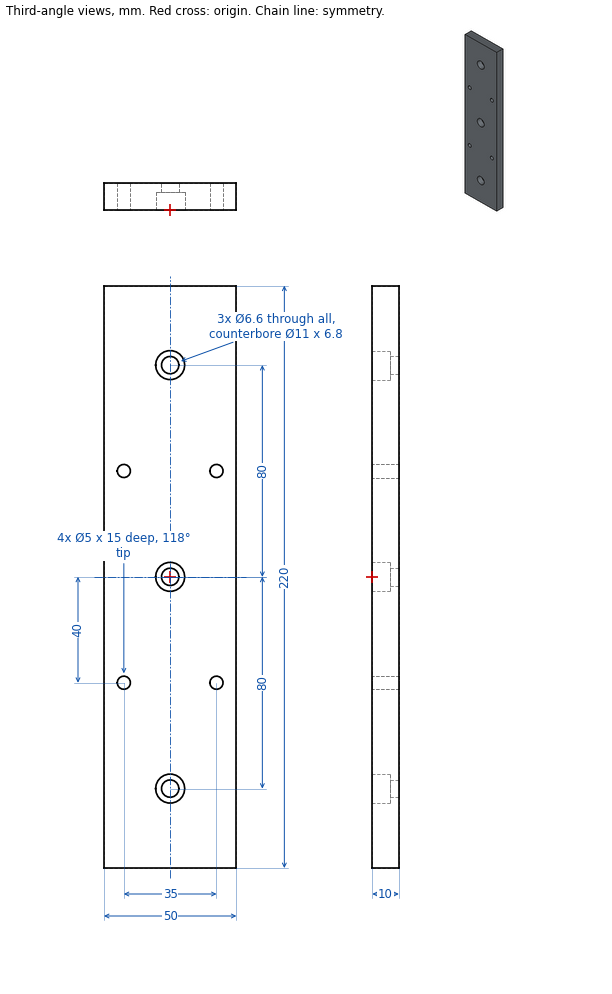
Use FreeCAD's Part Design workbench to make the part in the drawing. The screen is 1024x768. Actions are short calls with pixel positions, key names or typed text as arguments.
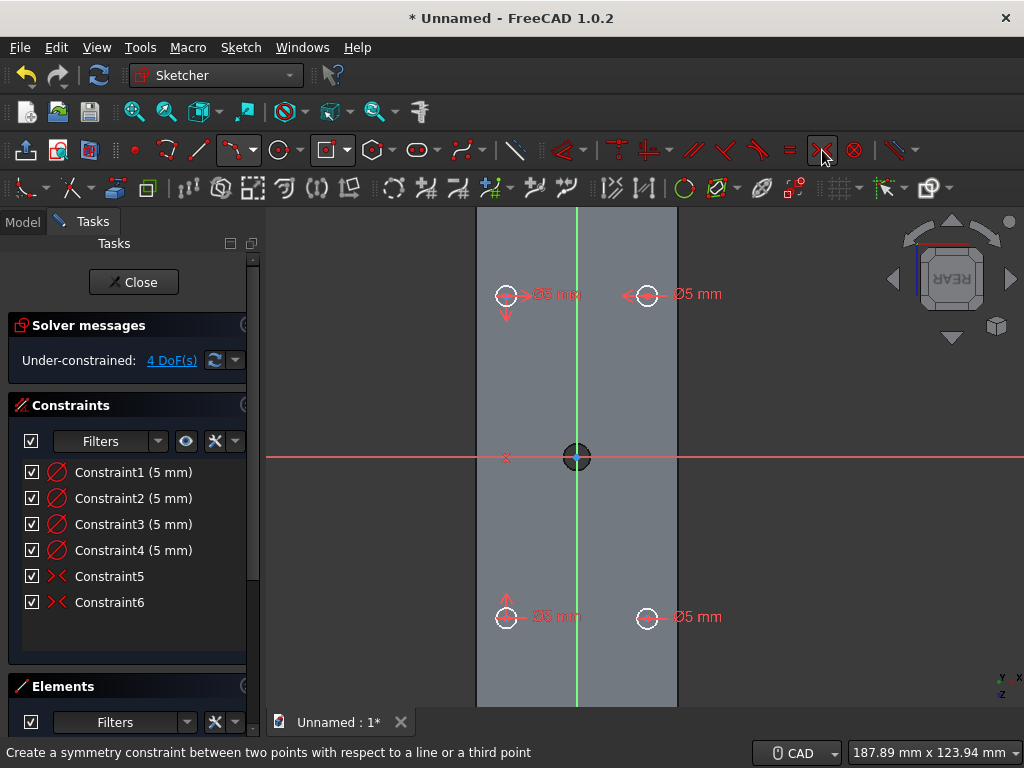
click(506, 618)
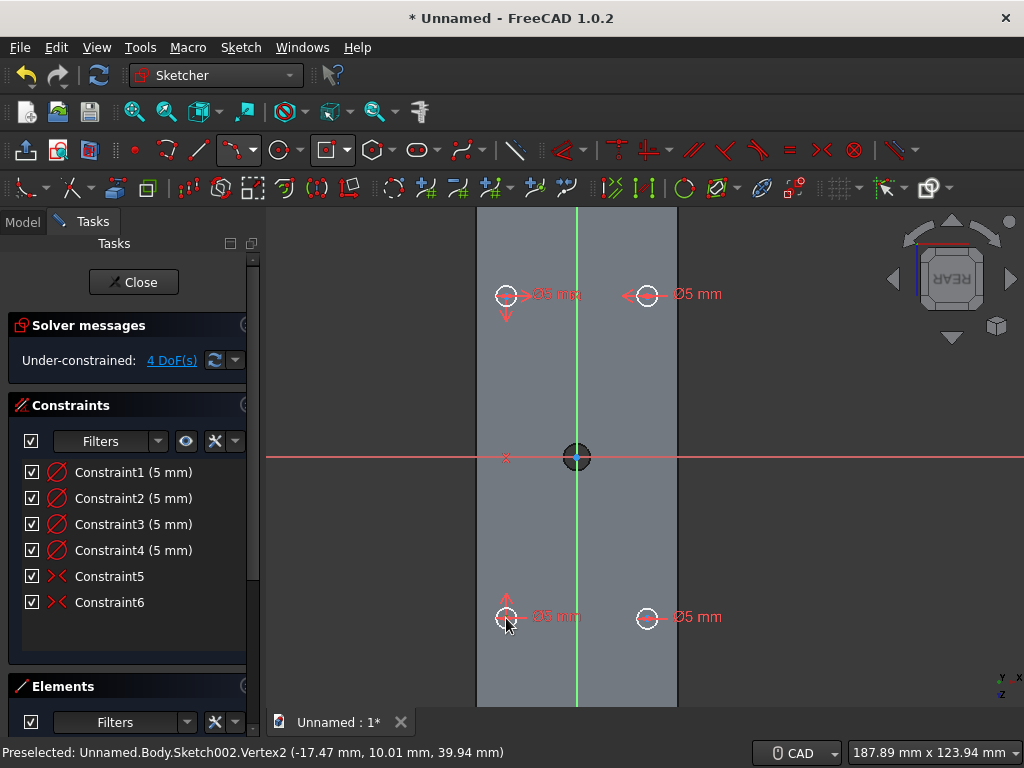
click(647, 619)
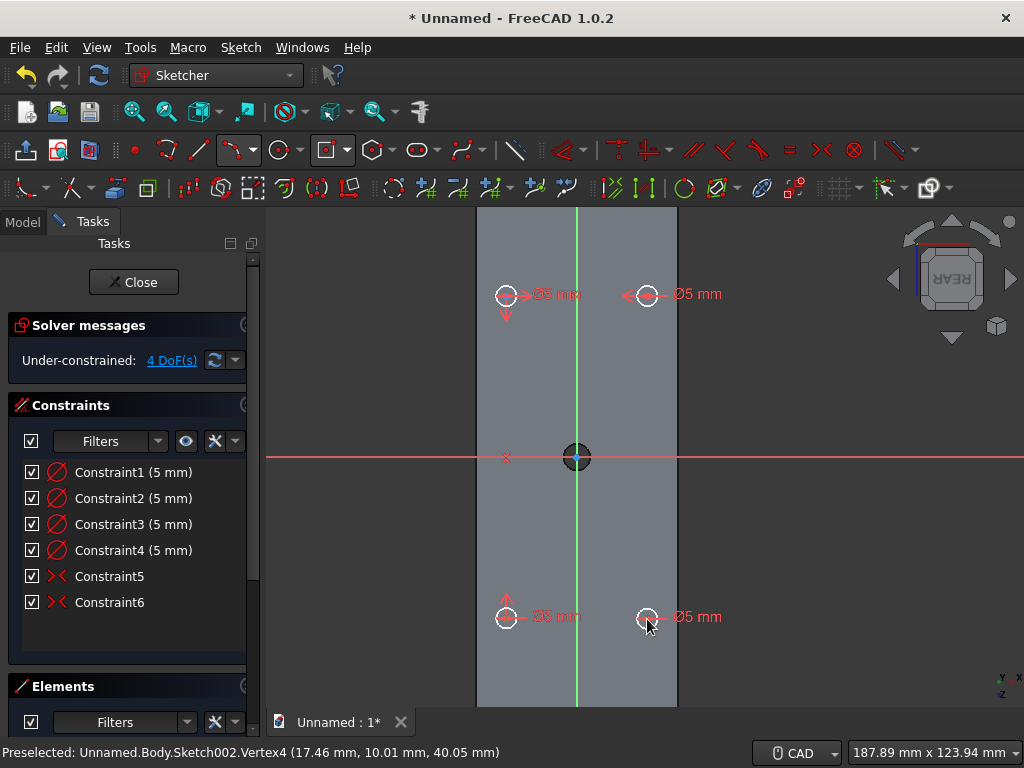
click(577, 647)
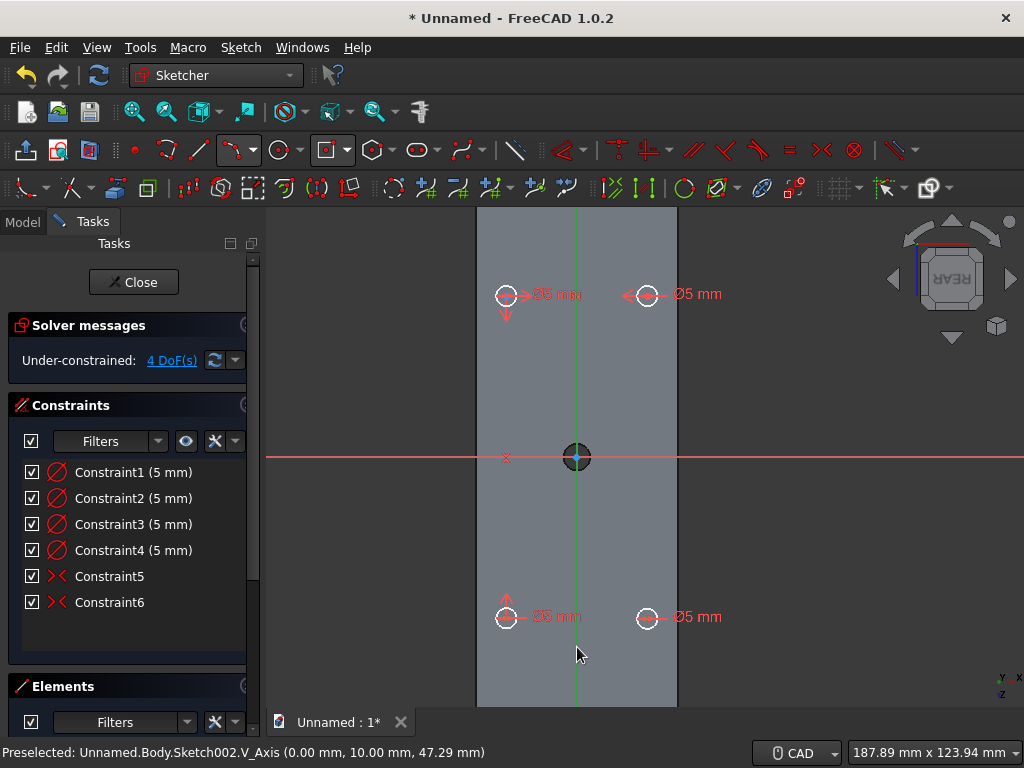
click(822, 150)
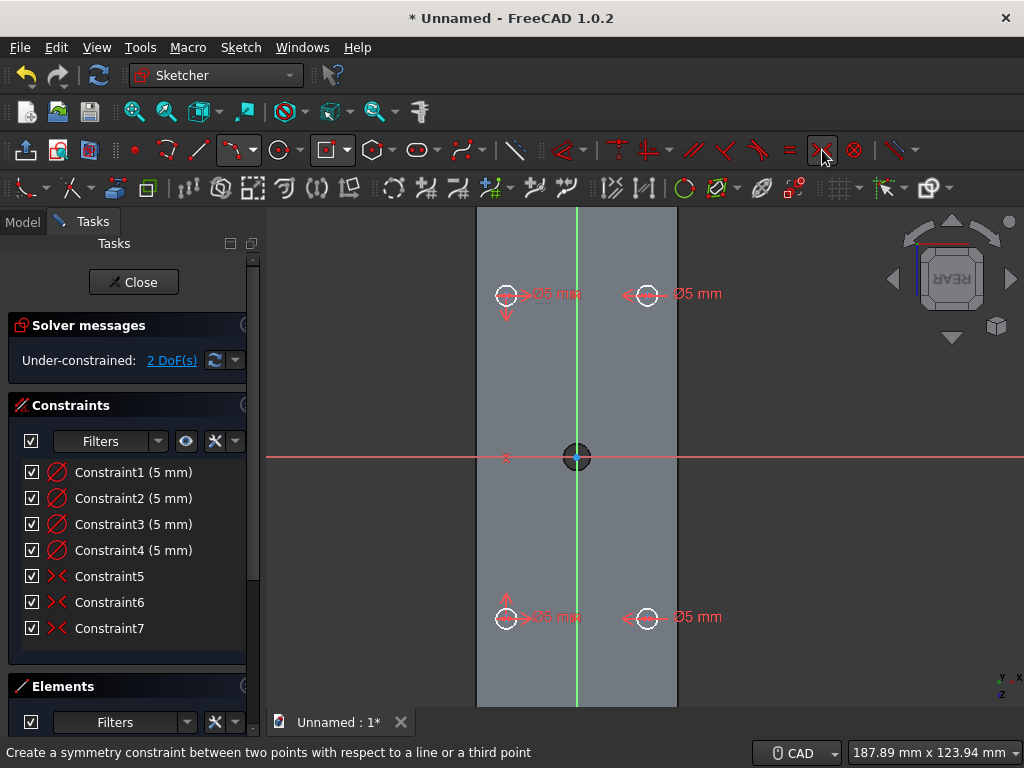
key(d)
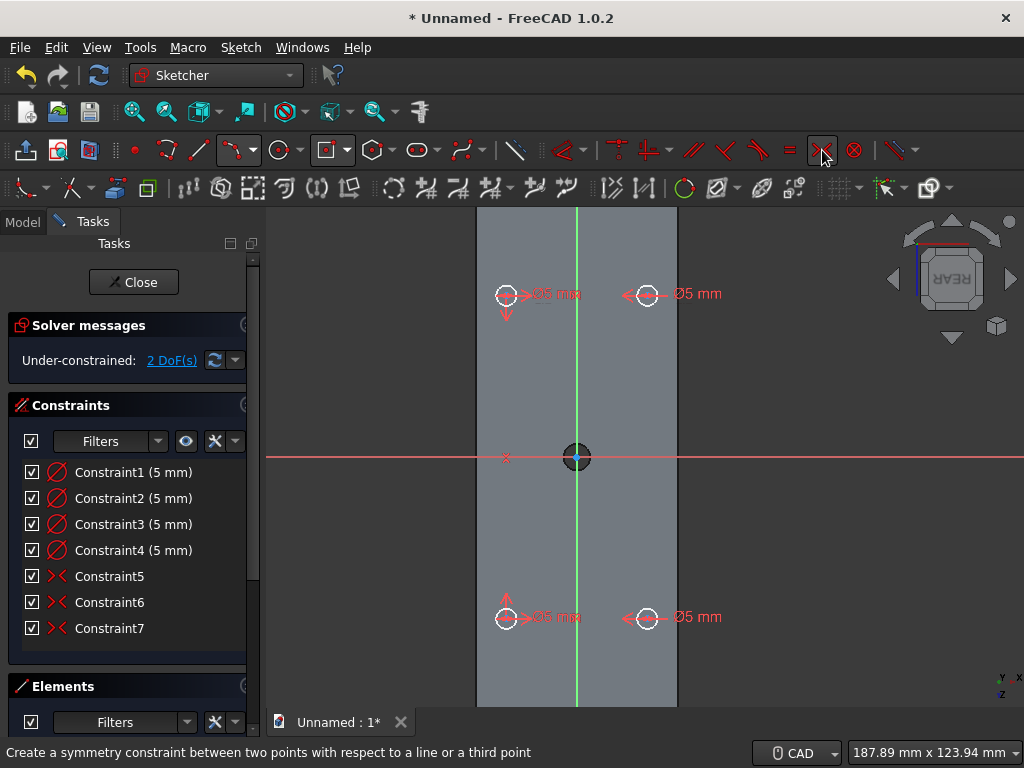
click(506, 296)
click(472, 376)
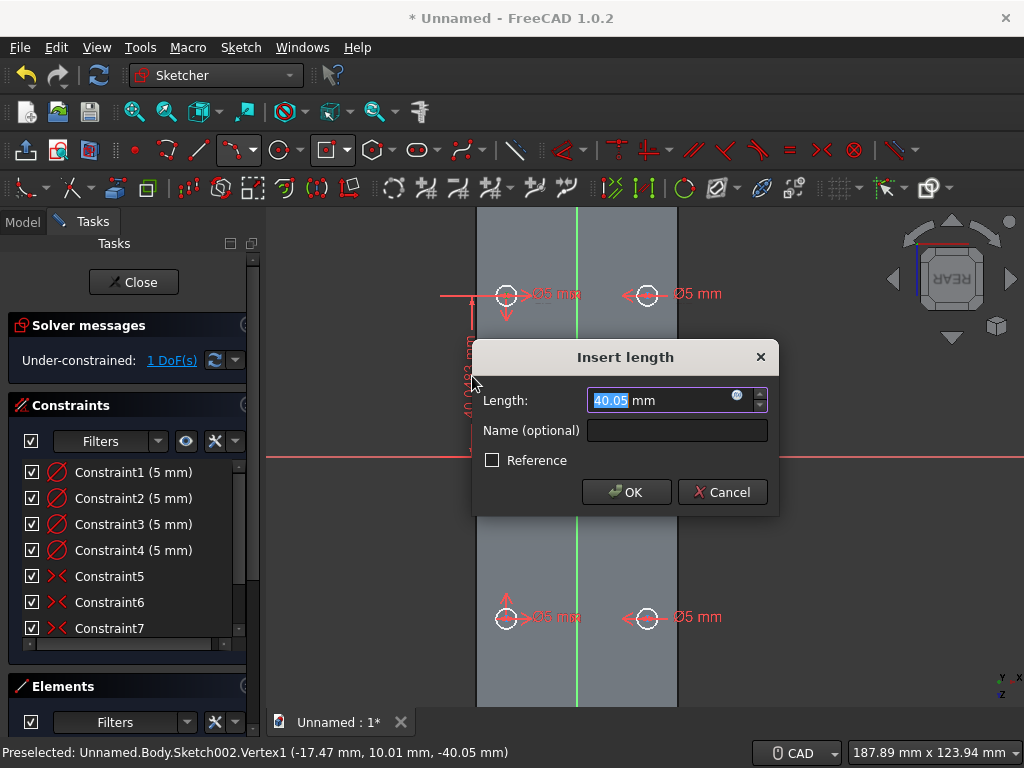
text(40)
key(Return)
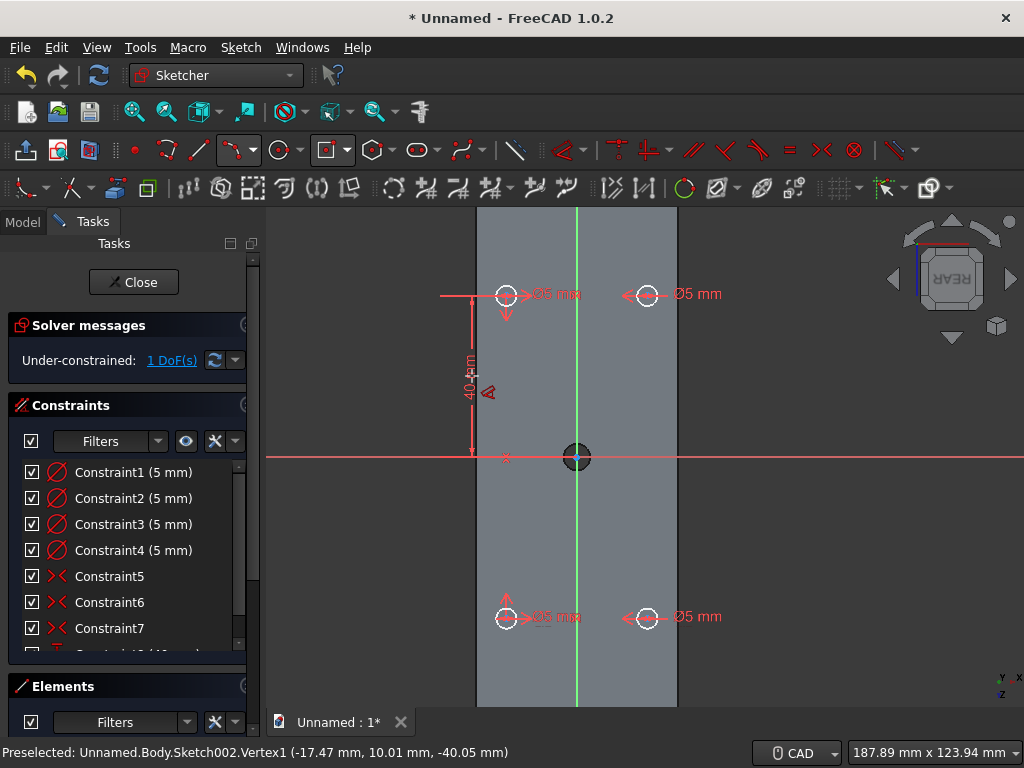
click(506, 296)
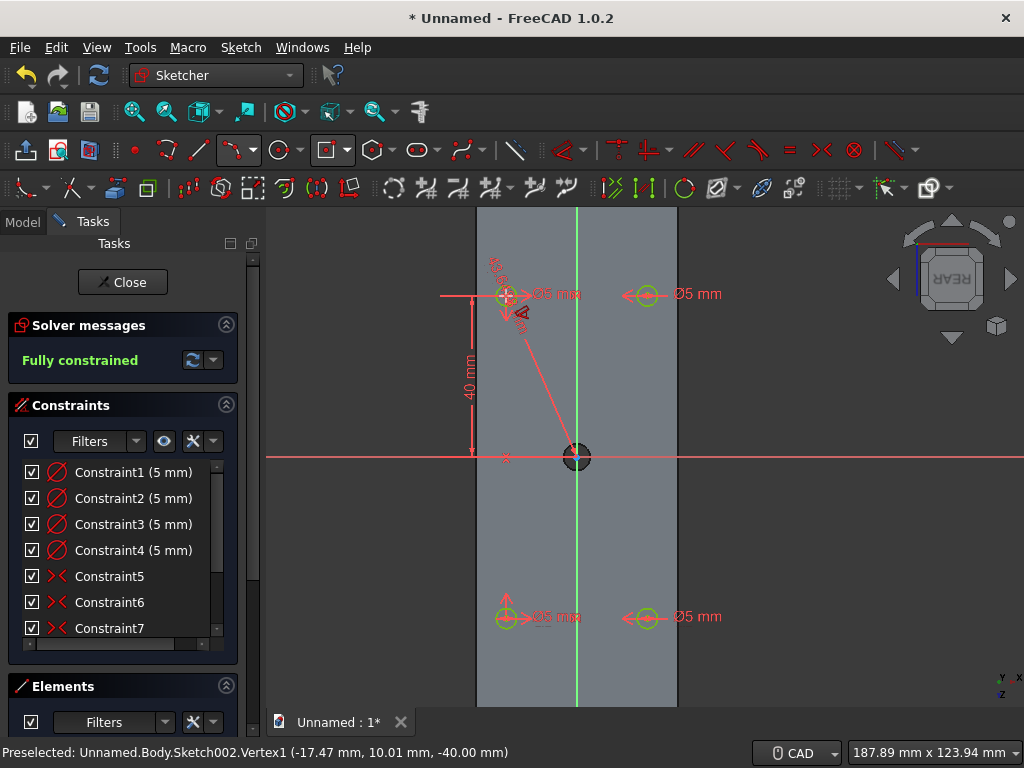
click(647, 296)
click(544, 262)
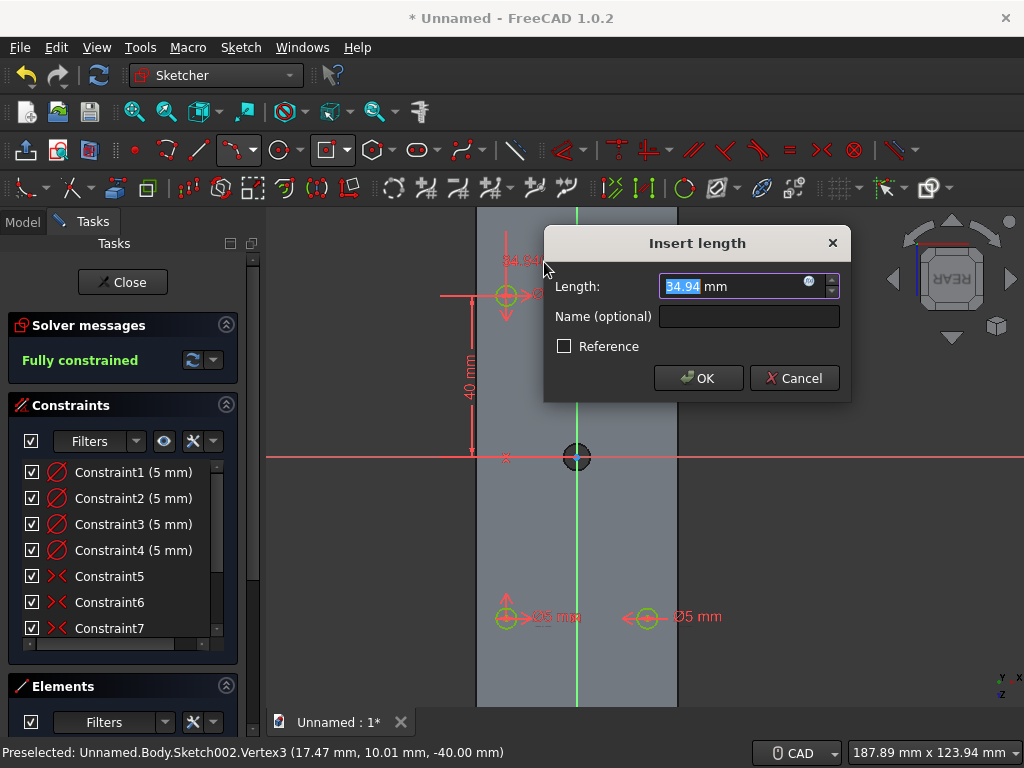
text(35)
key(Return)
key(Escape)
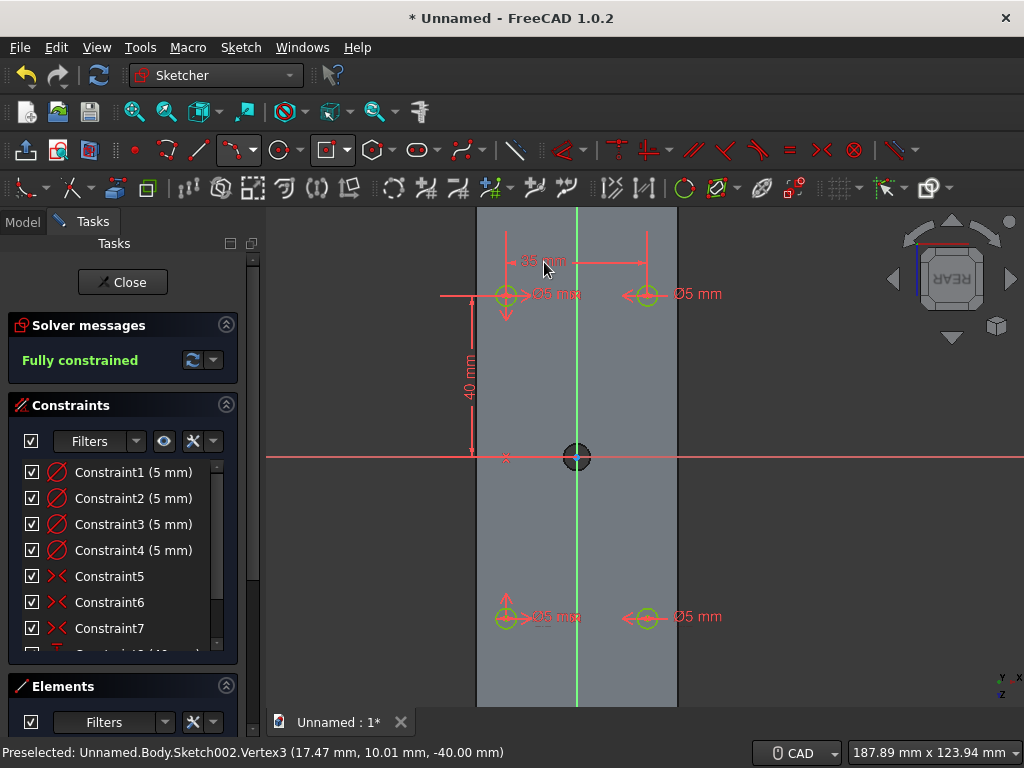
click(123, 282)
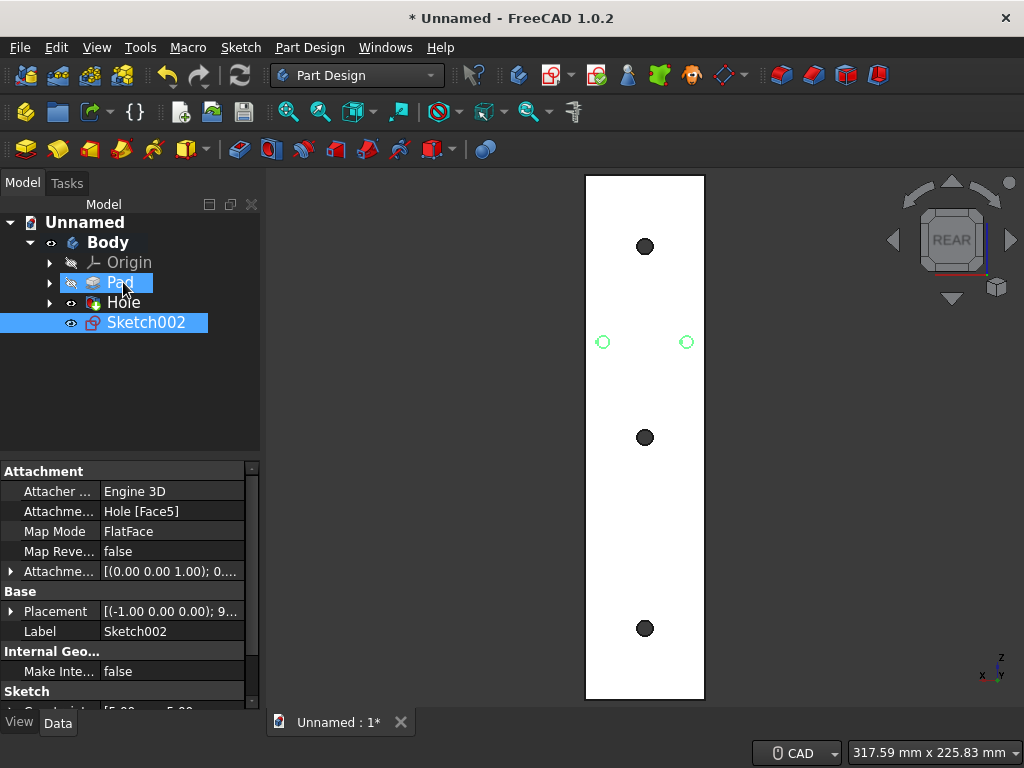
click(272, 150)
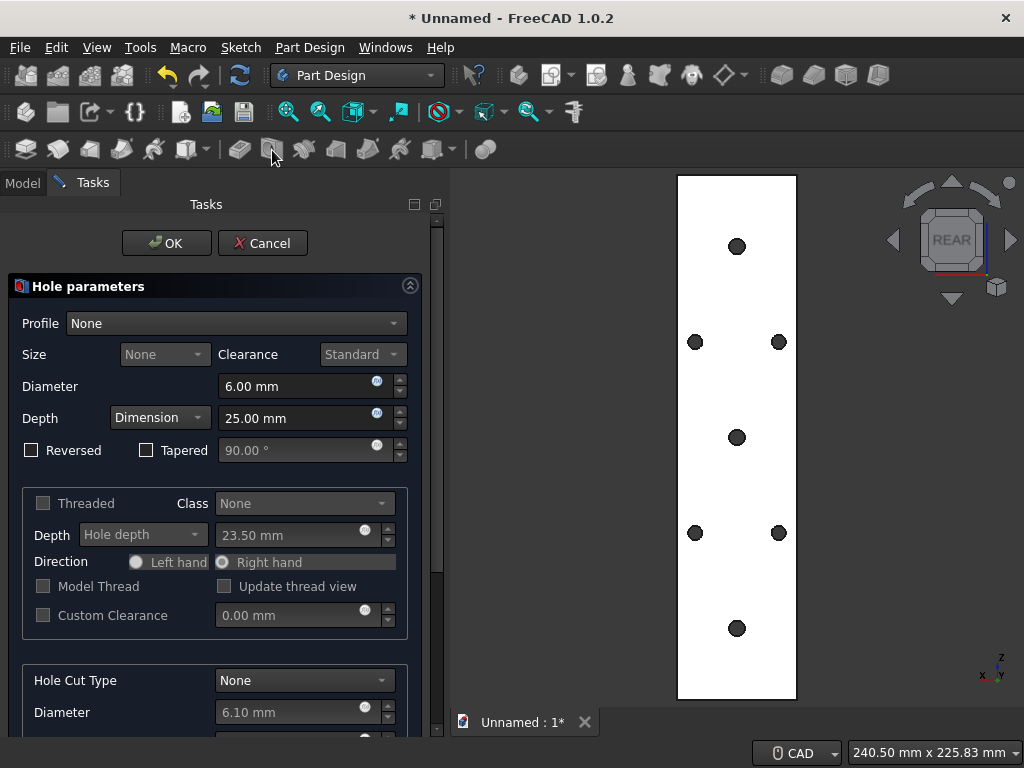
triple_click(305, 386)